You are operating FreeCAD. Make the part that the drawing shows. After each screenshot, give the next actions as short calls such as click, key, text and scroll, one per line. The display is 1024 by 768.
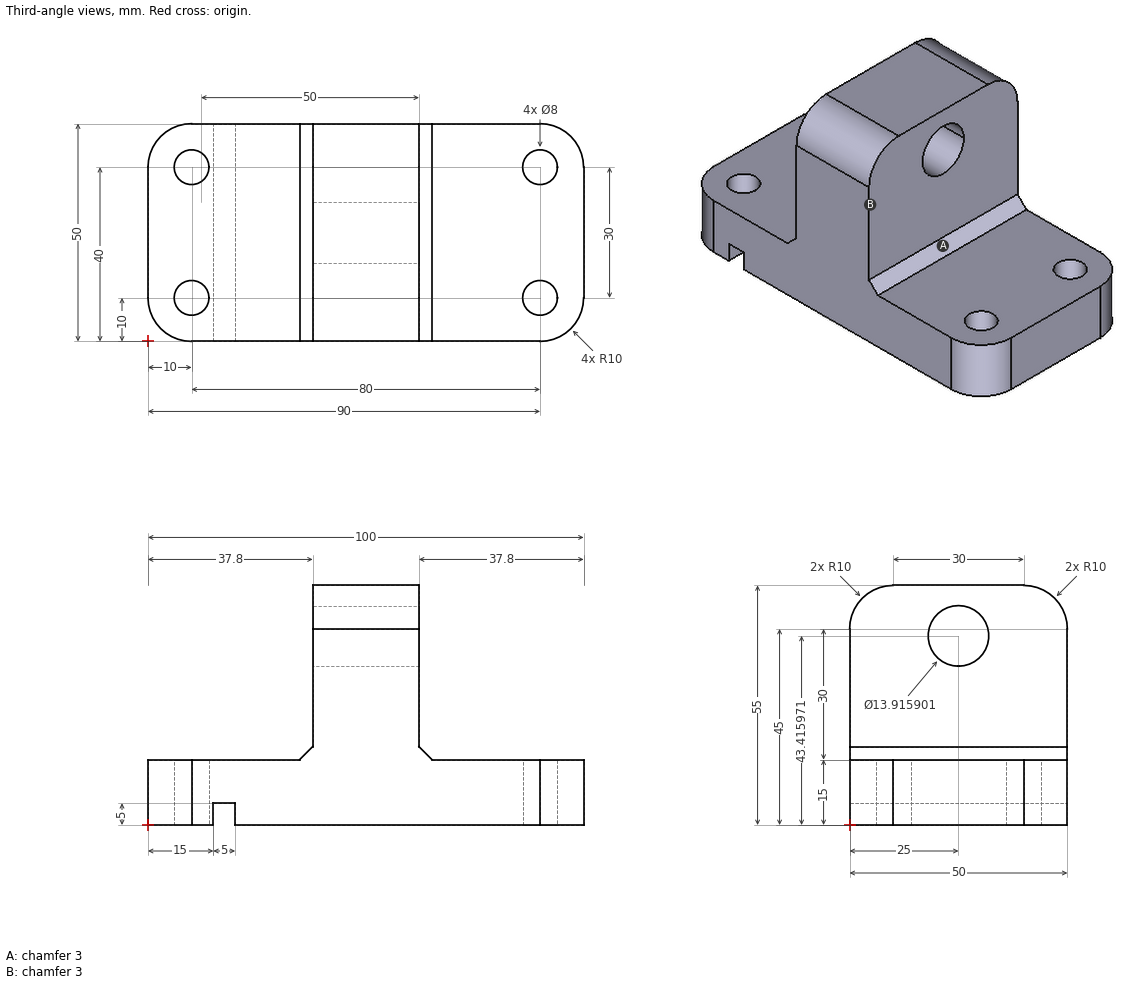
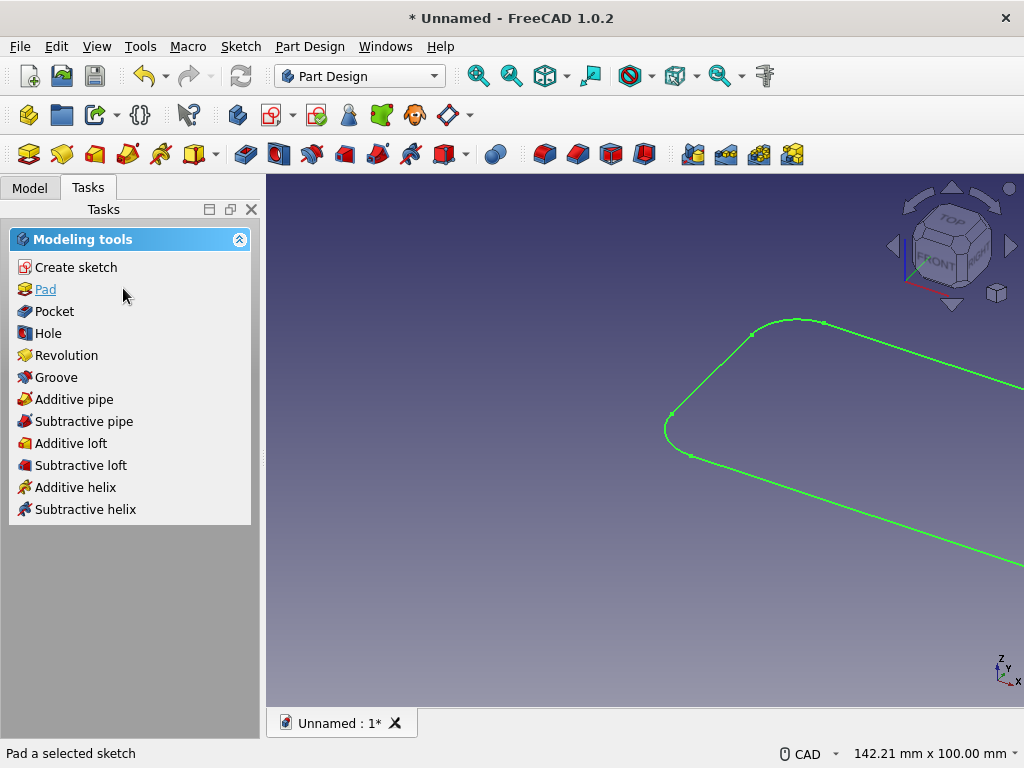
click(29, 154)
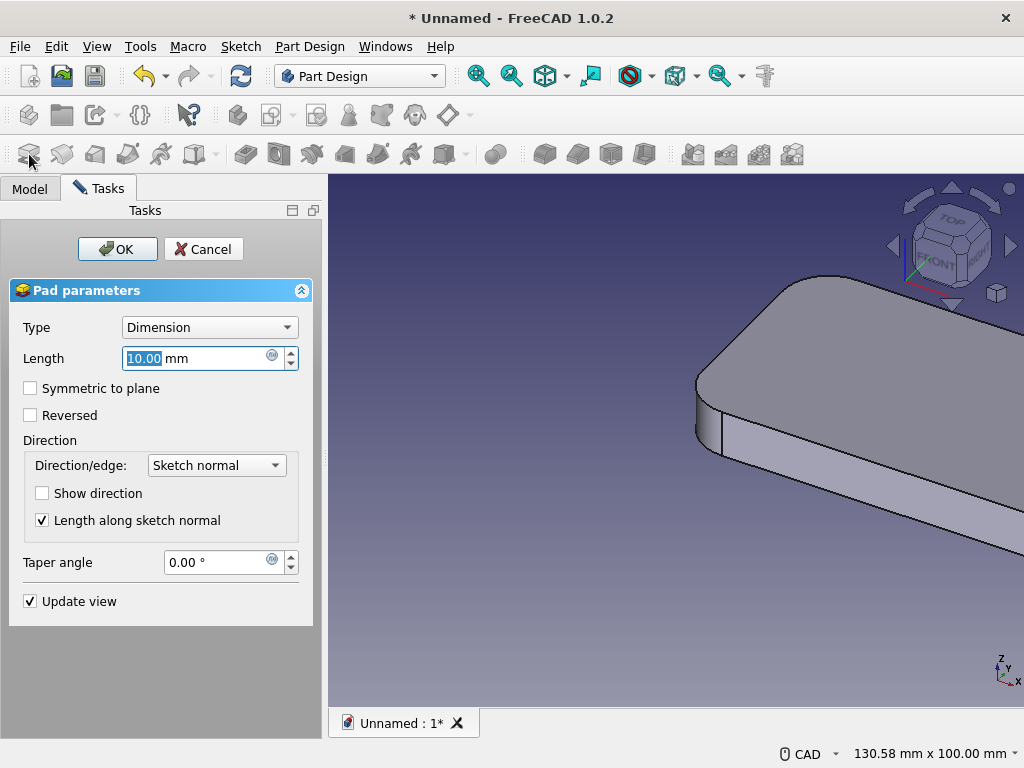
text(15)
key(Tab)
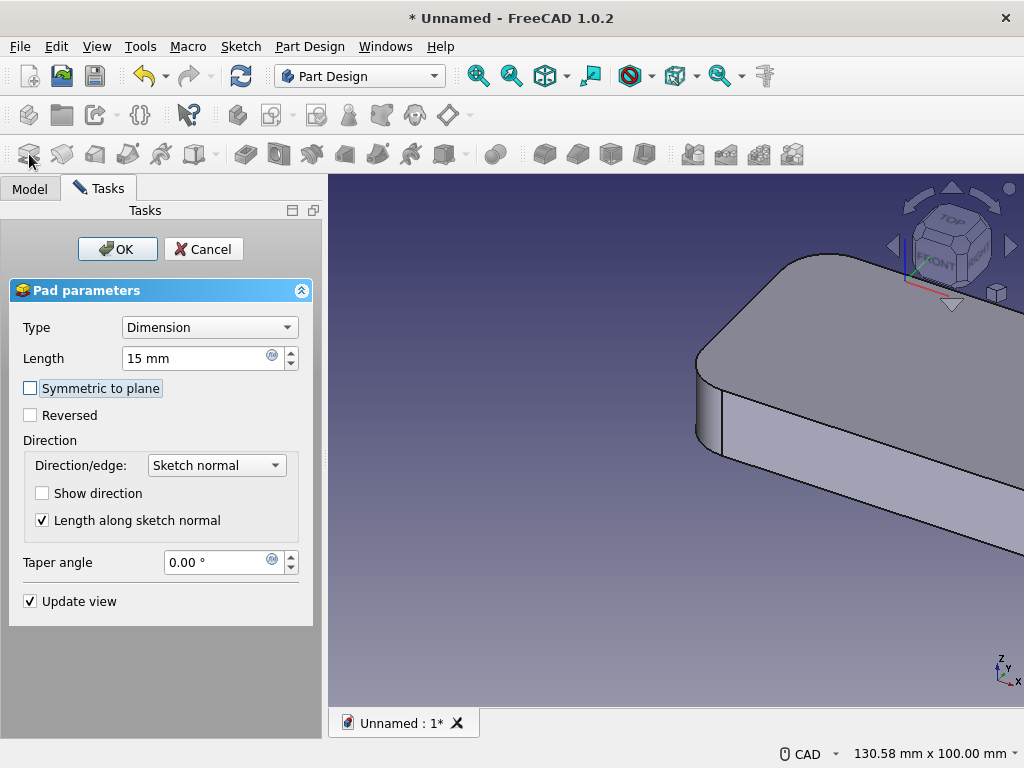
click(118, 249)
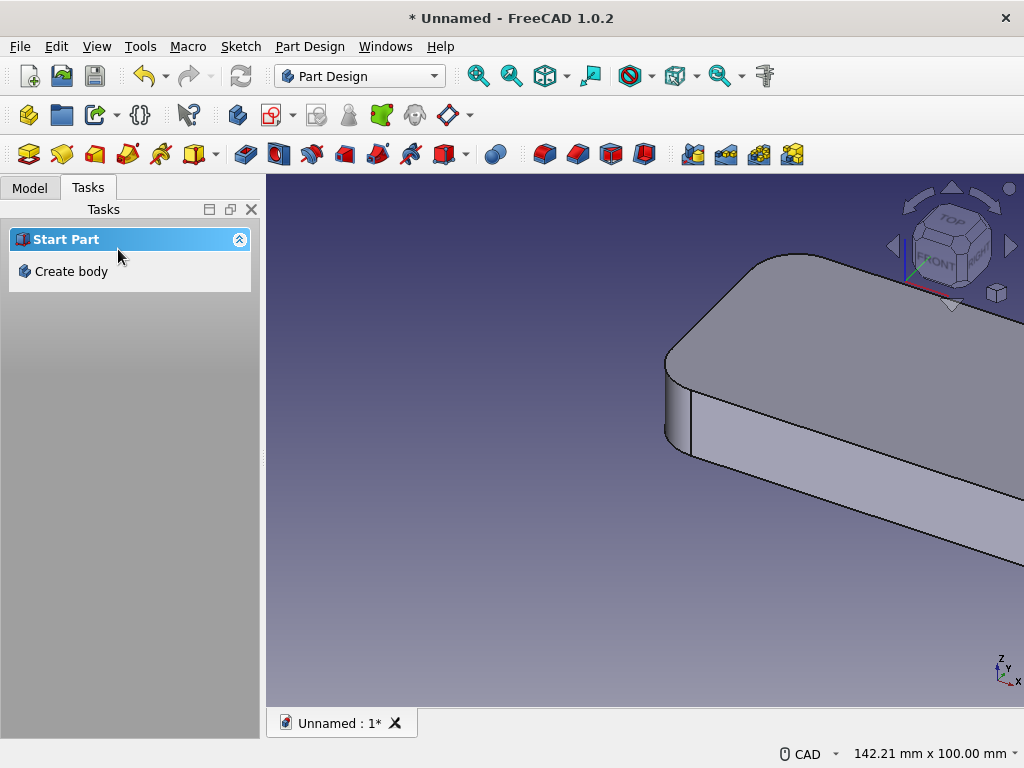
click(479, 76)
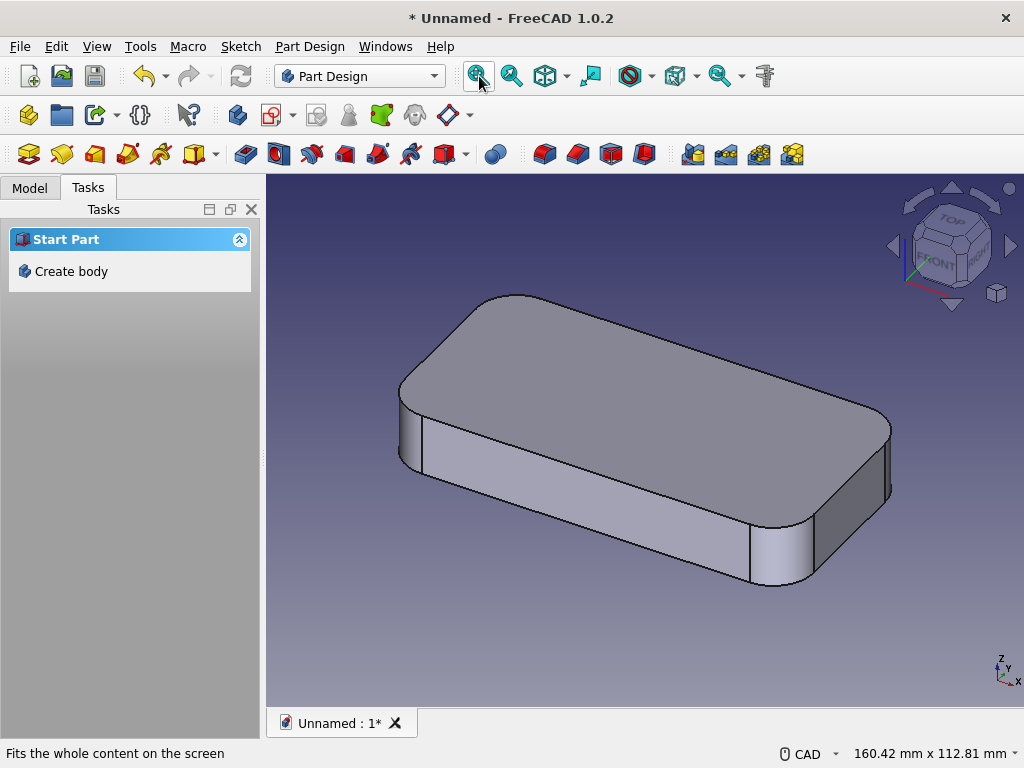
click(860, 497)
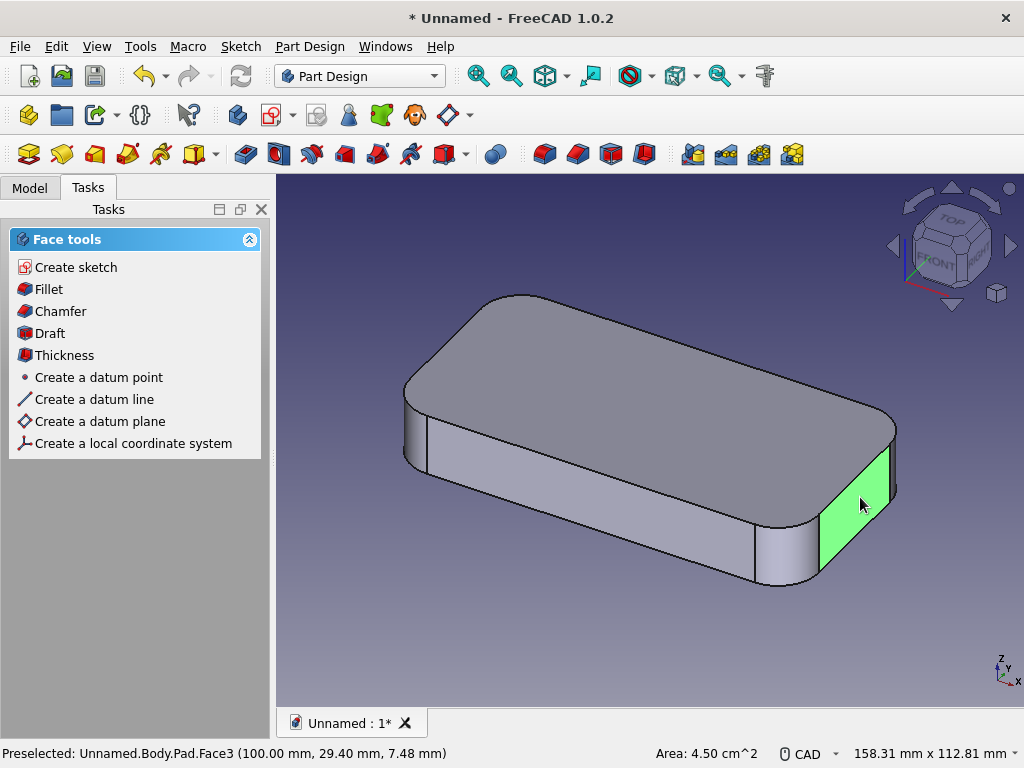
click(270, 116)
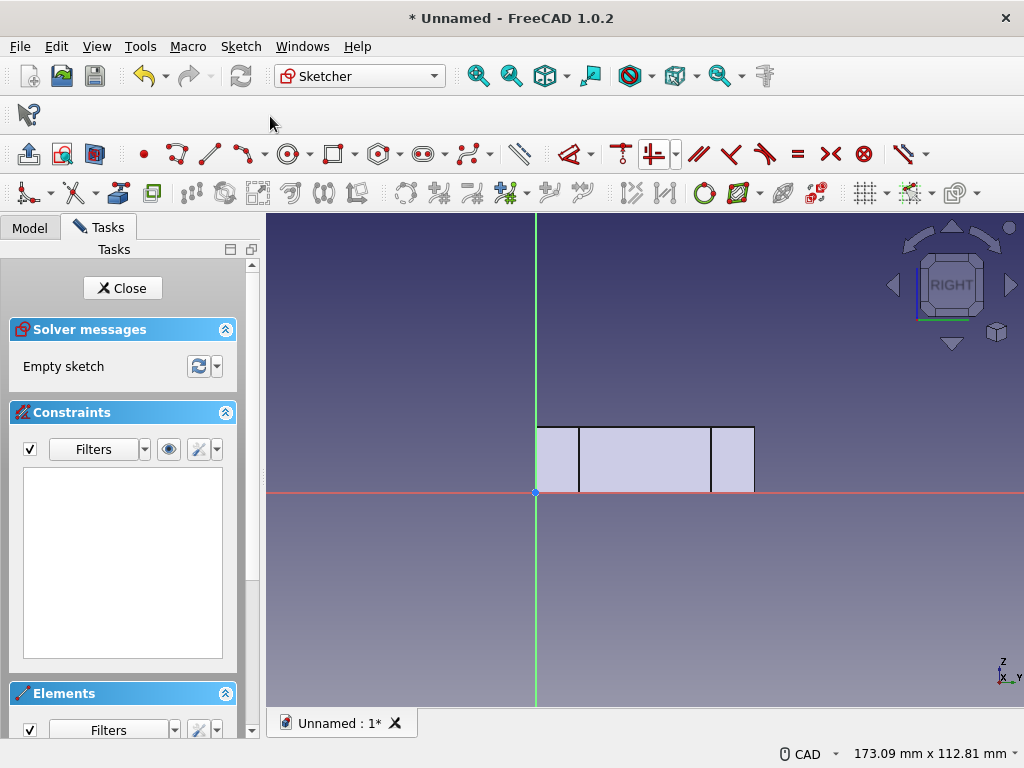
scroll(294, 679, down, 1)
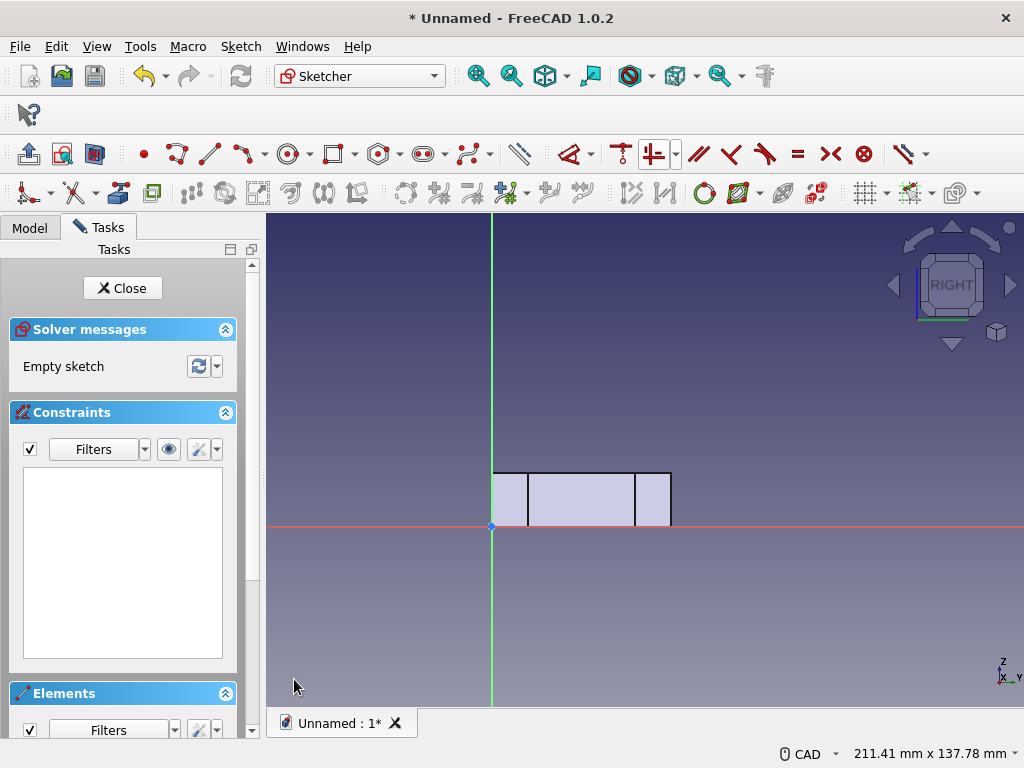
scroll(591, 363, up, 2)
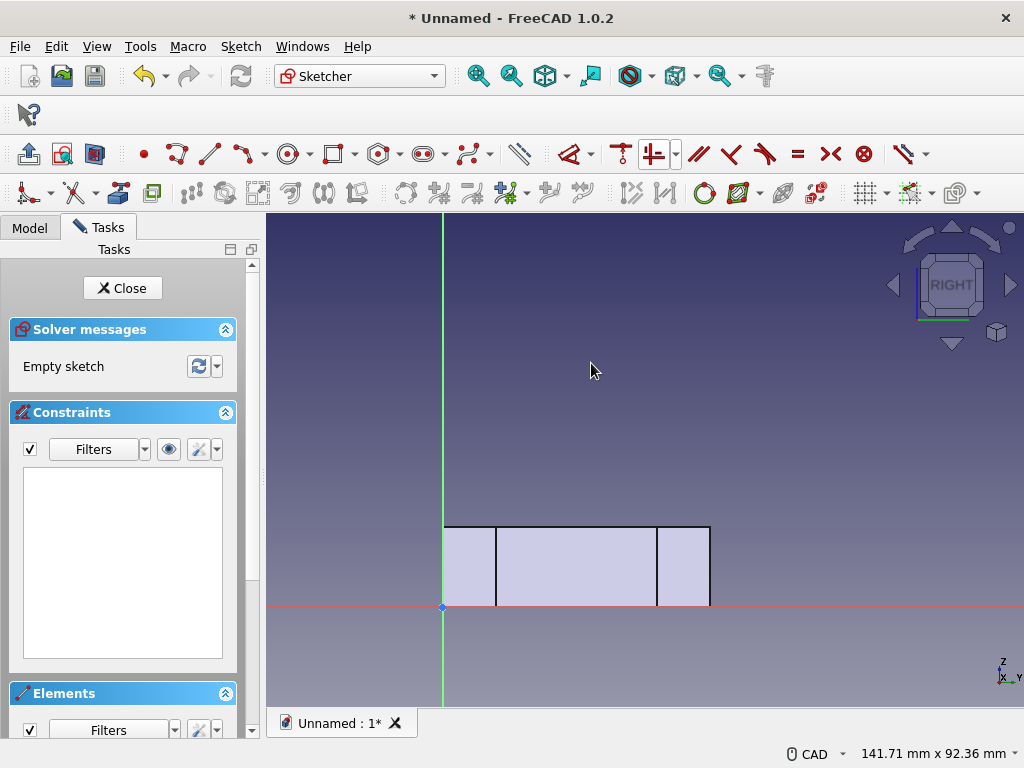
click(210, 154)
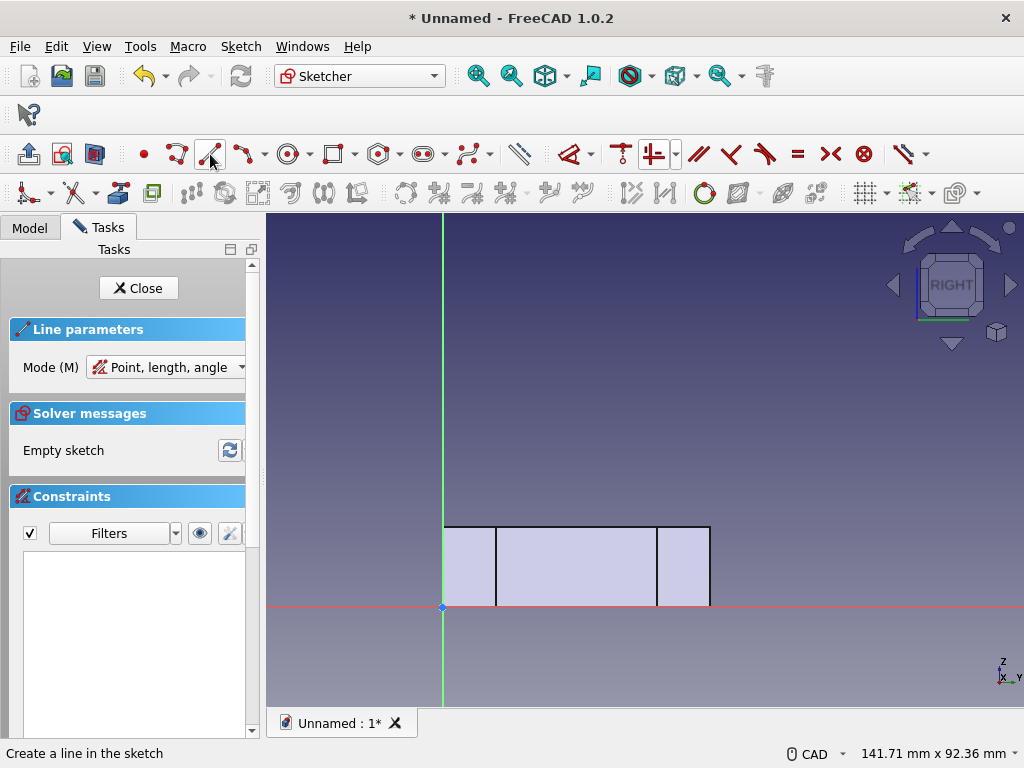
click(657, 313)
click(496, 313)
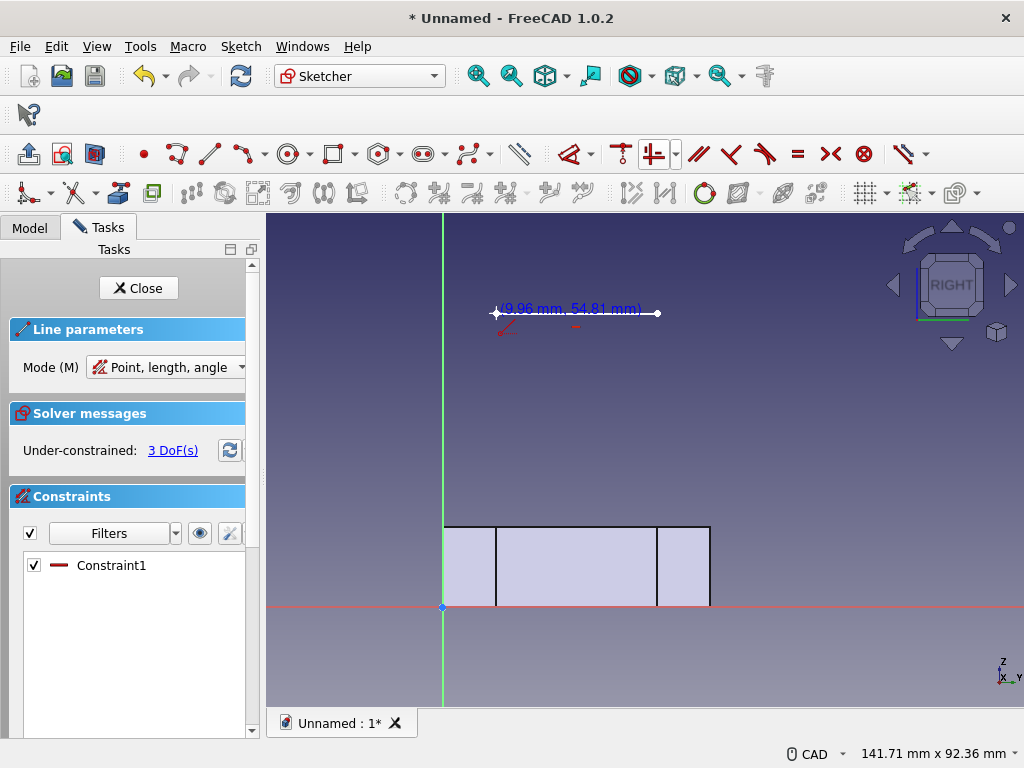
click(177, 154)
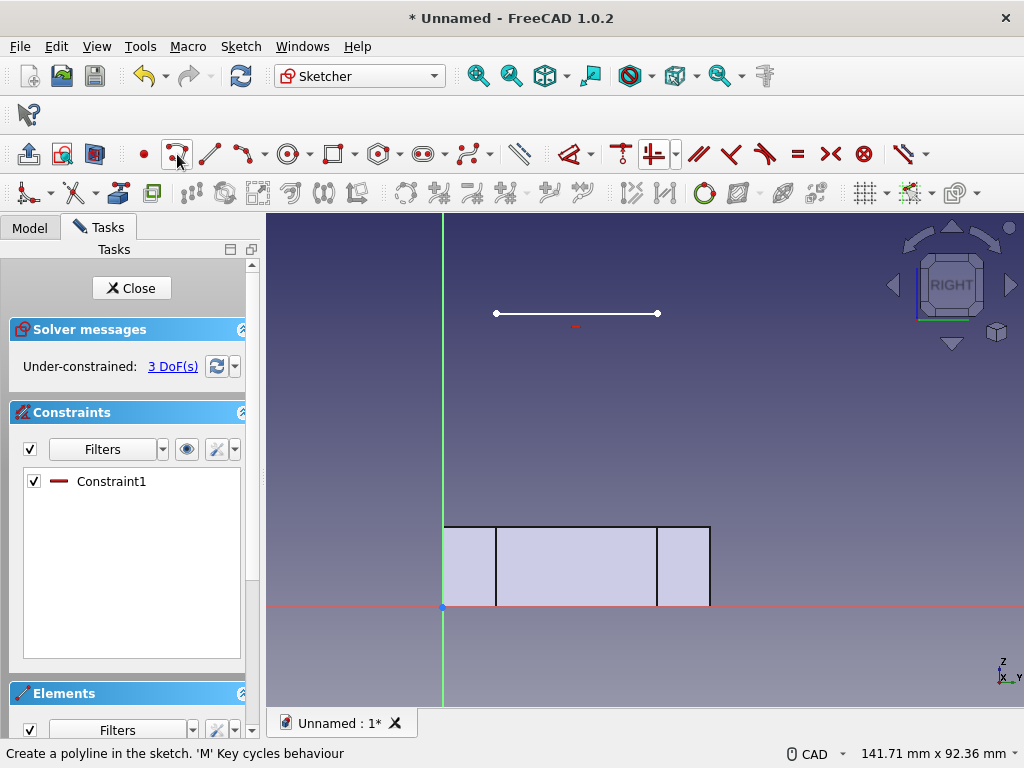
click(443, 366)
click(452, 527)
click(710, 527)
click(710, 366)
right_click(710, 366)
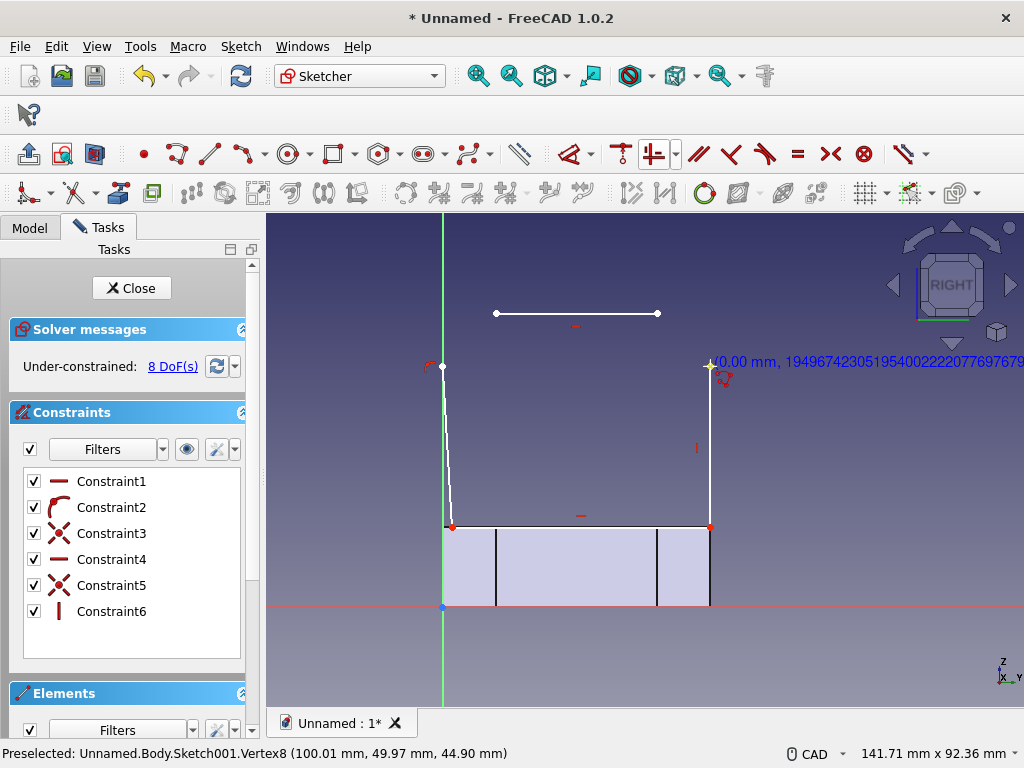
click(242, 154)